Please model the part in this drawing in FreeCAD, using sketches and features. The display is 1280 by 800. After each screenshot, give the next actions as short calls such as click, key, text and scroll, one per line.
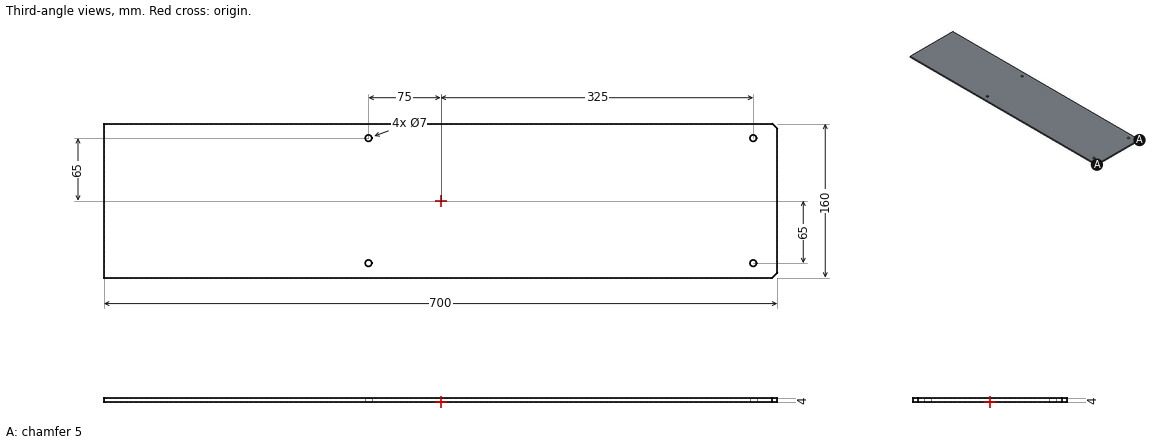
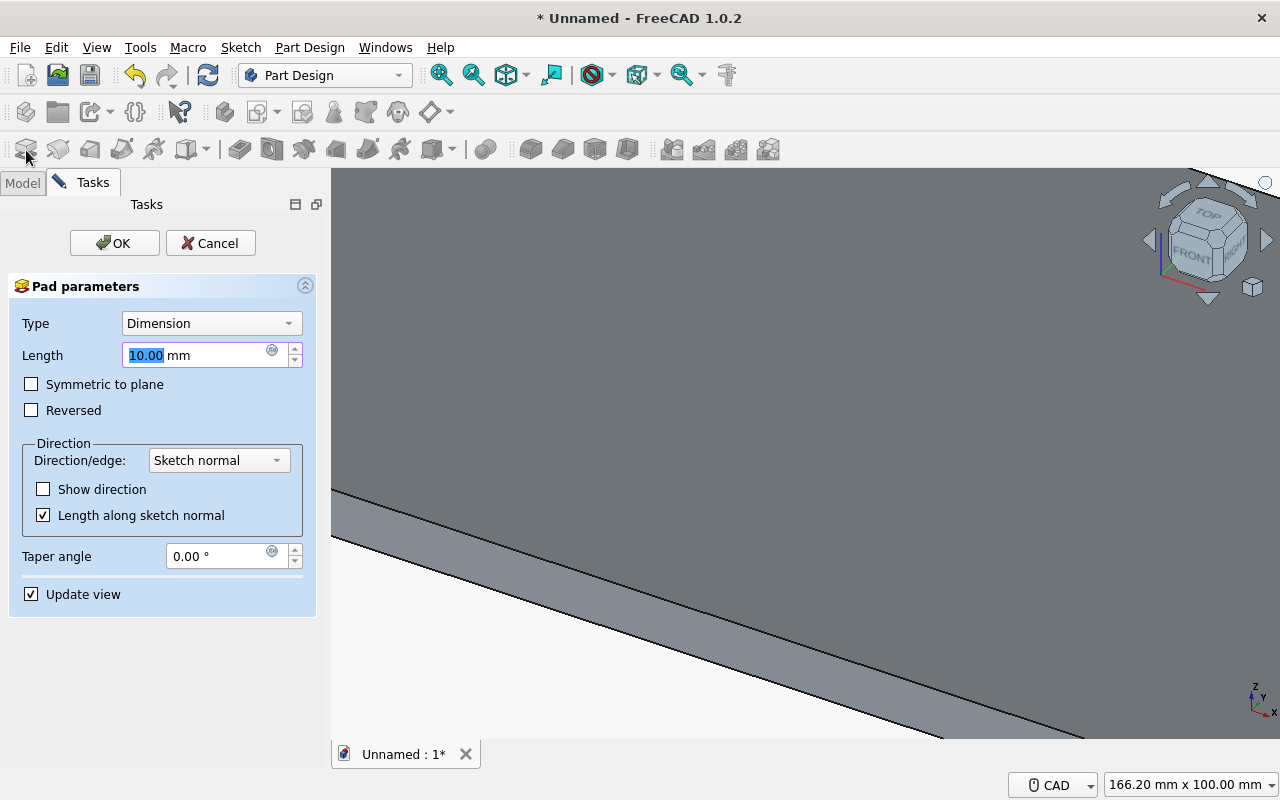
text(4)
key(Tab)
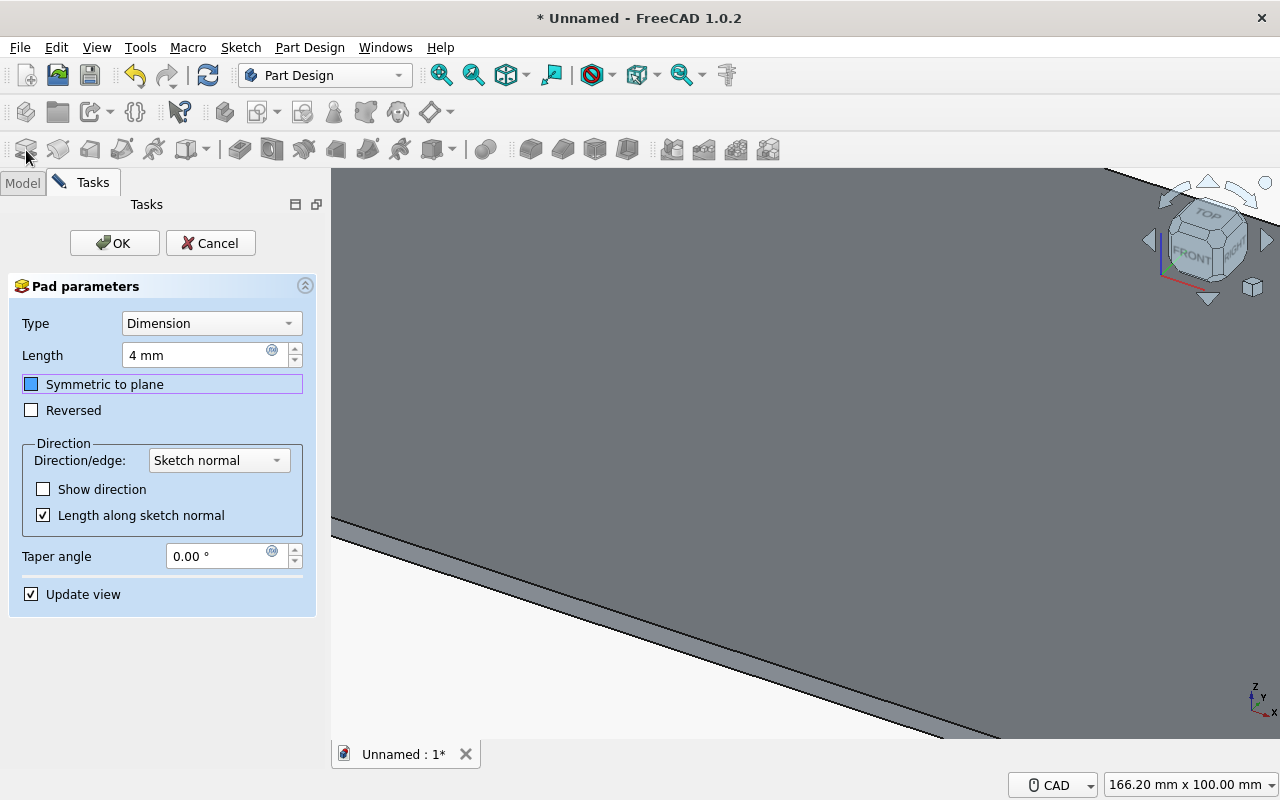
click(115, 243)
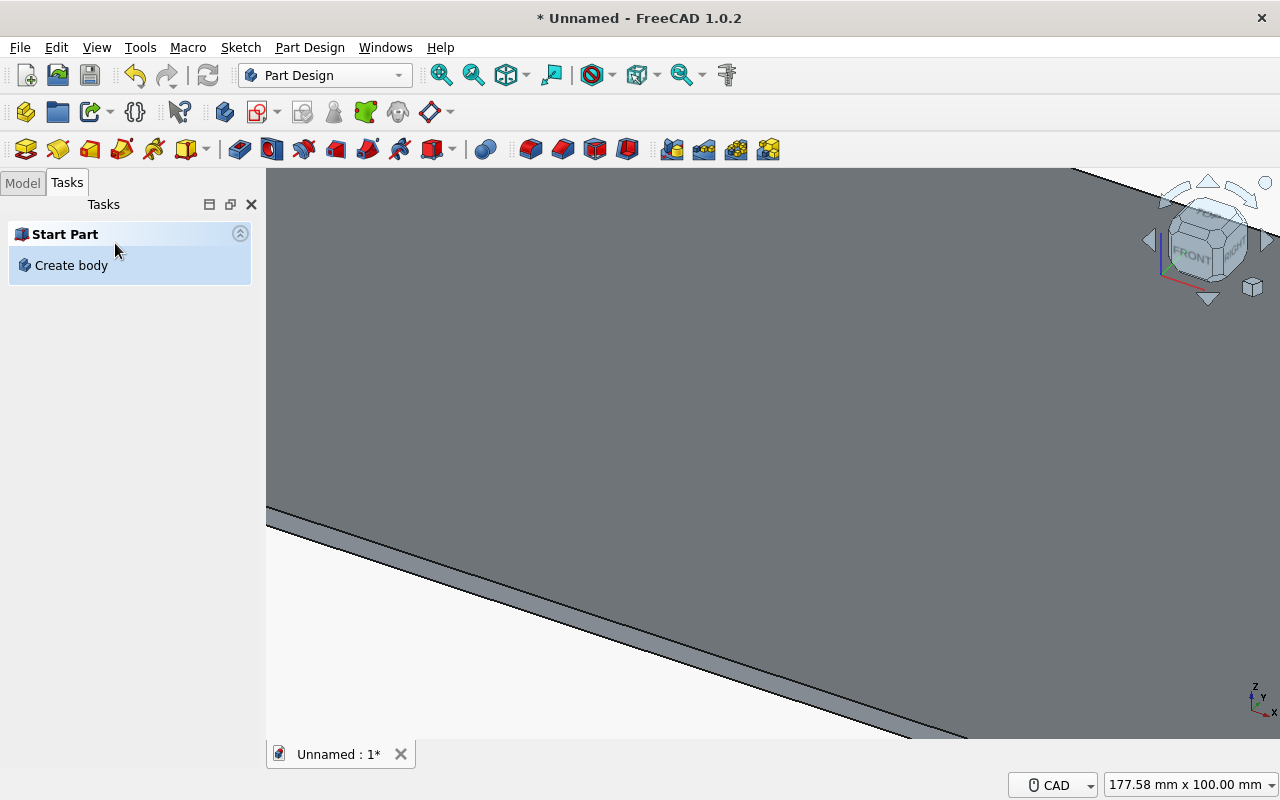
click(442, 76)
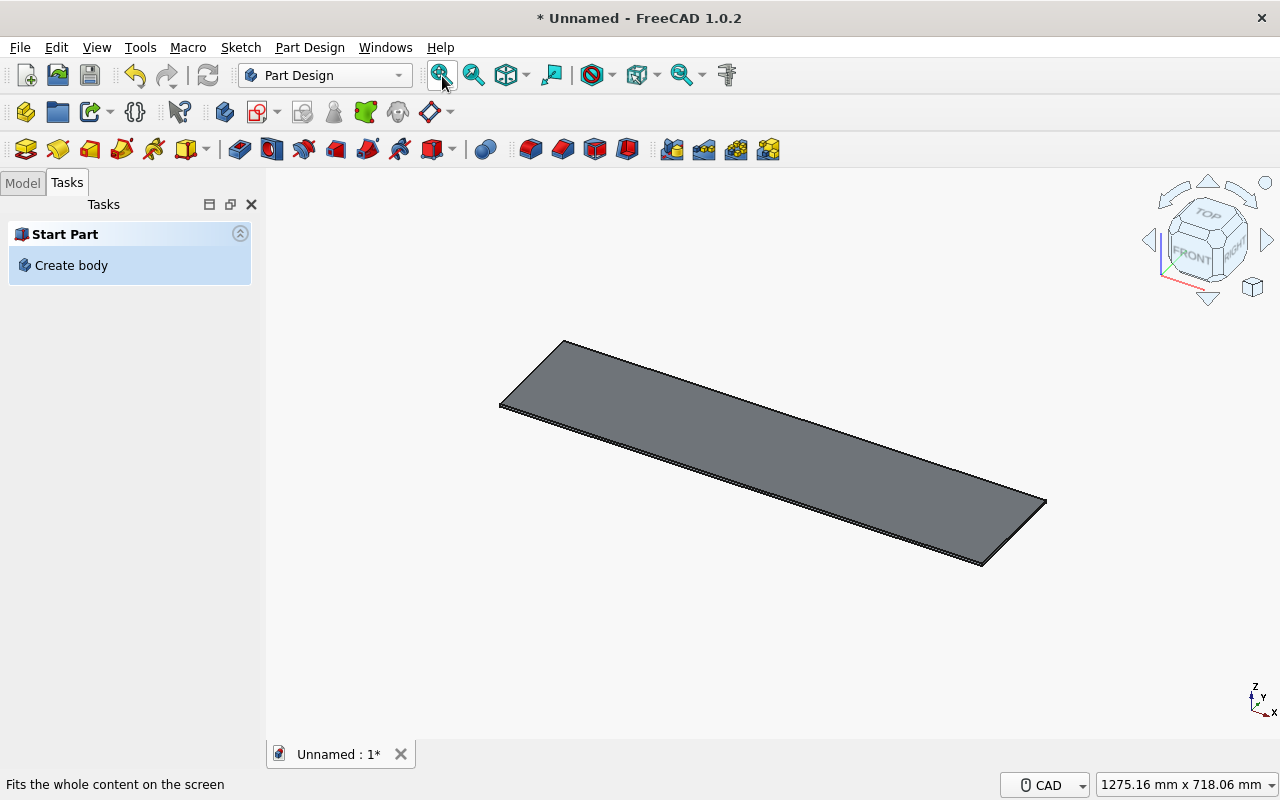
click(911, 497)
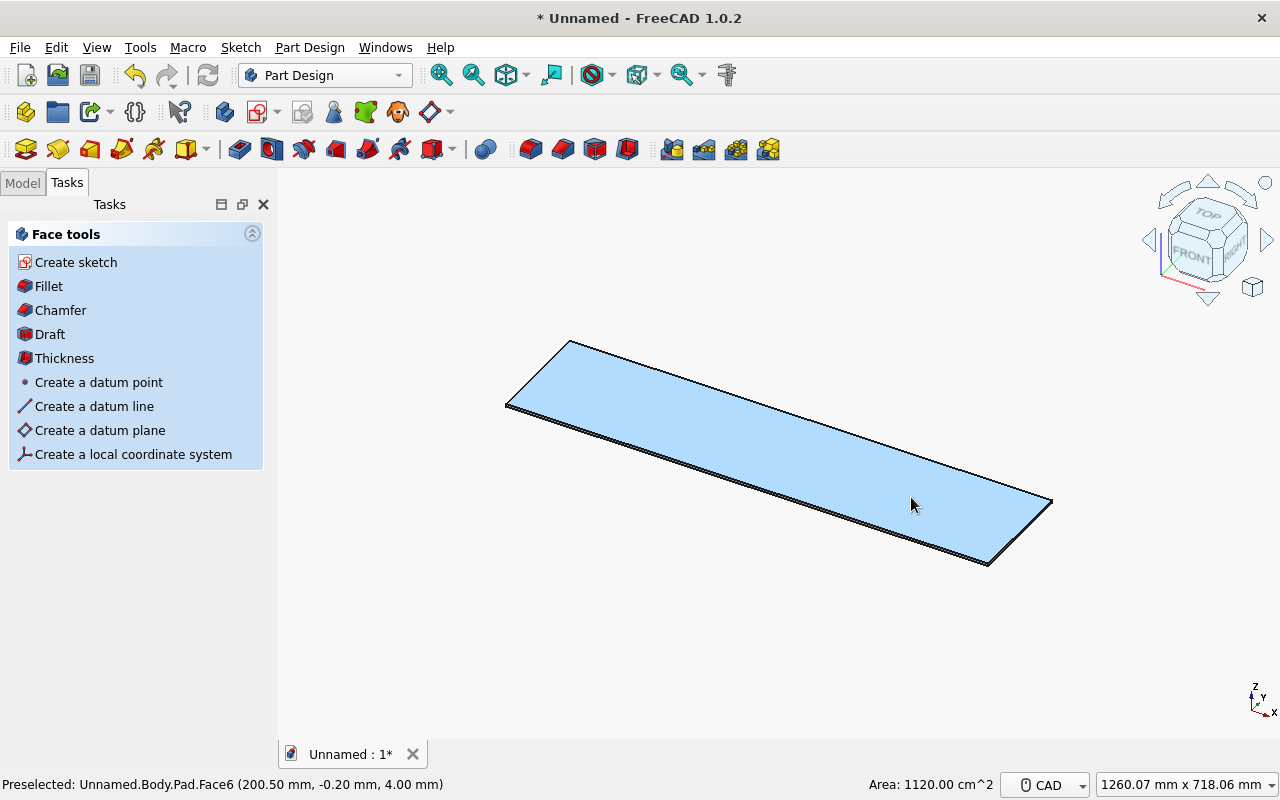
click(258, 112)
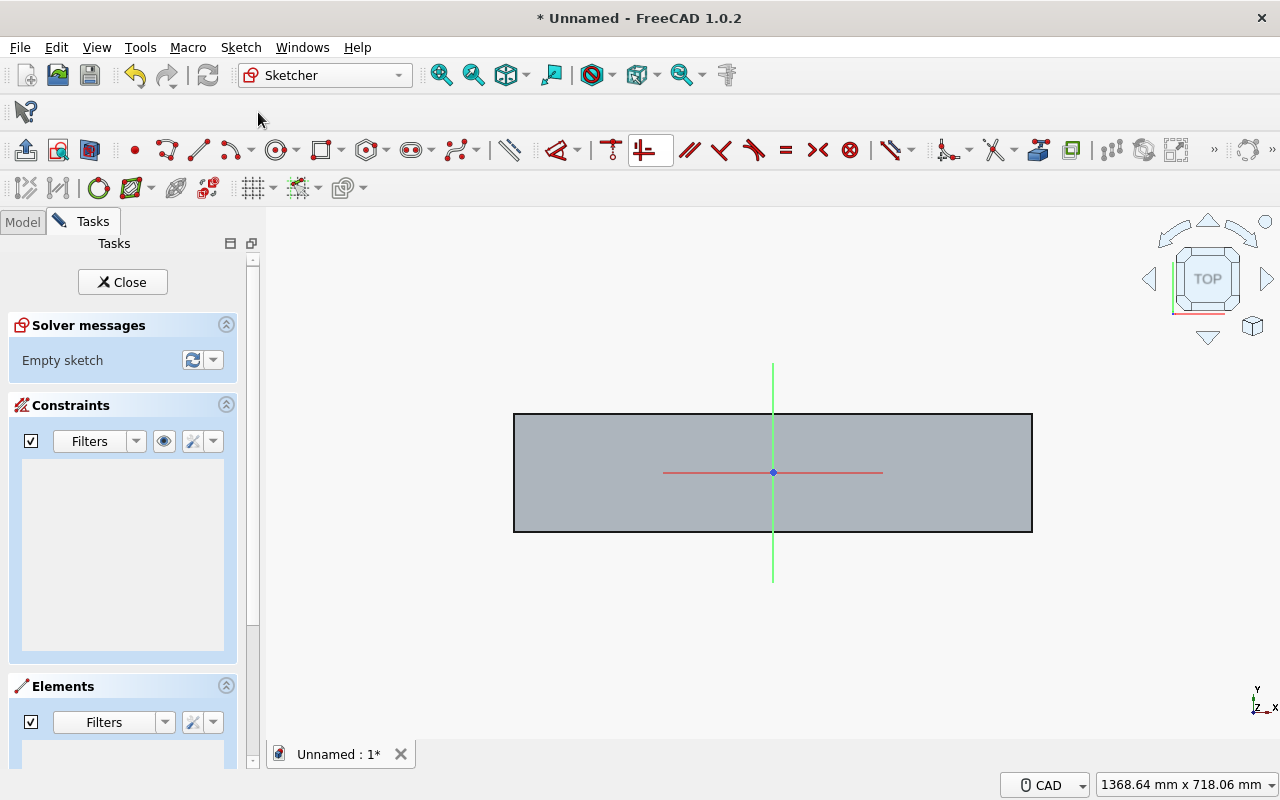
scroll(1062, 473, up, 3)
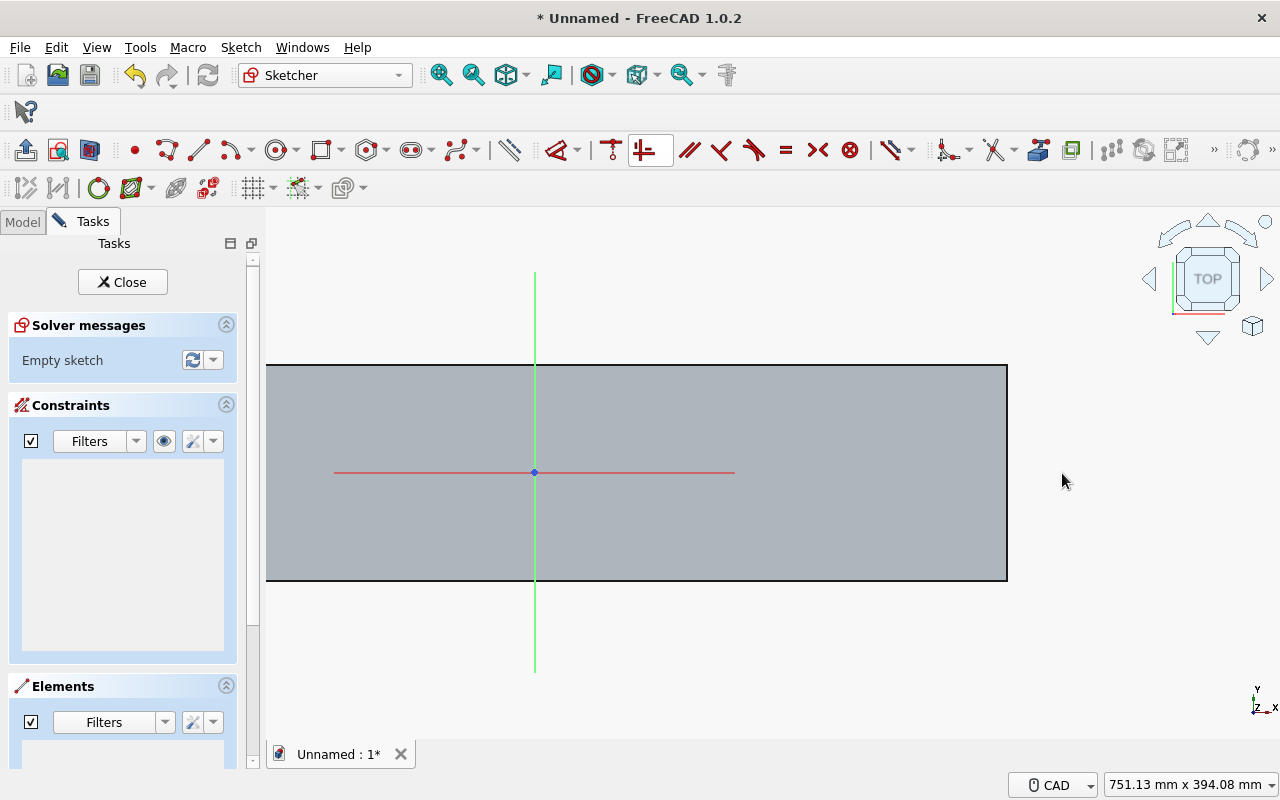
click(276, 150)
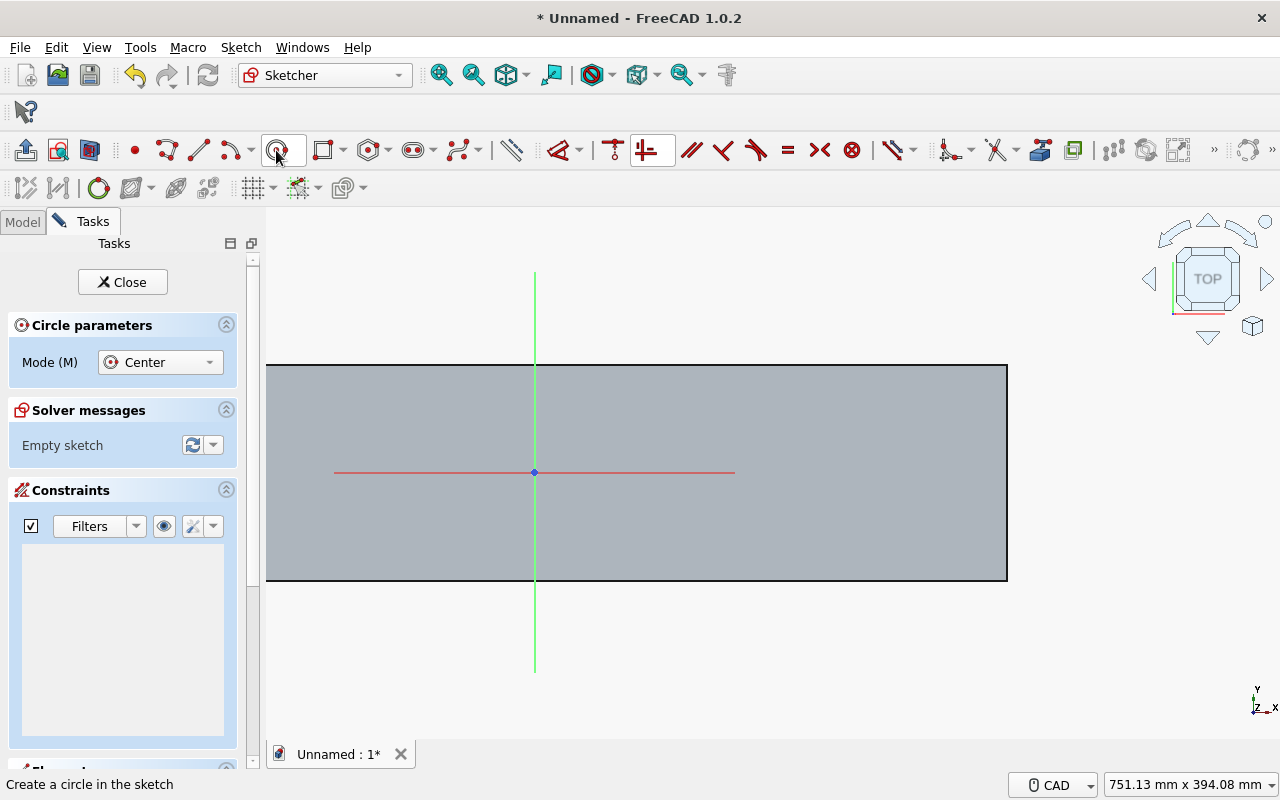
scroll(434, 385, up, 8)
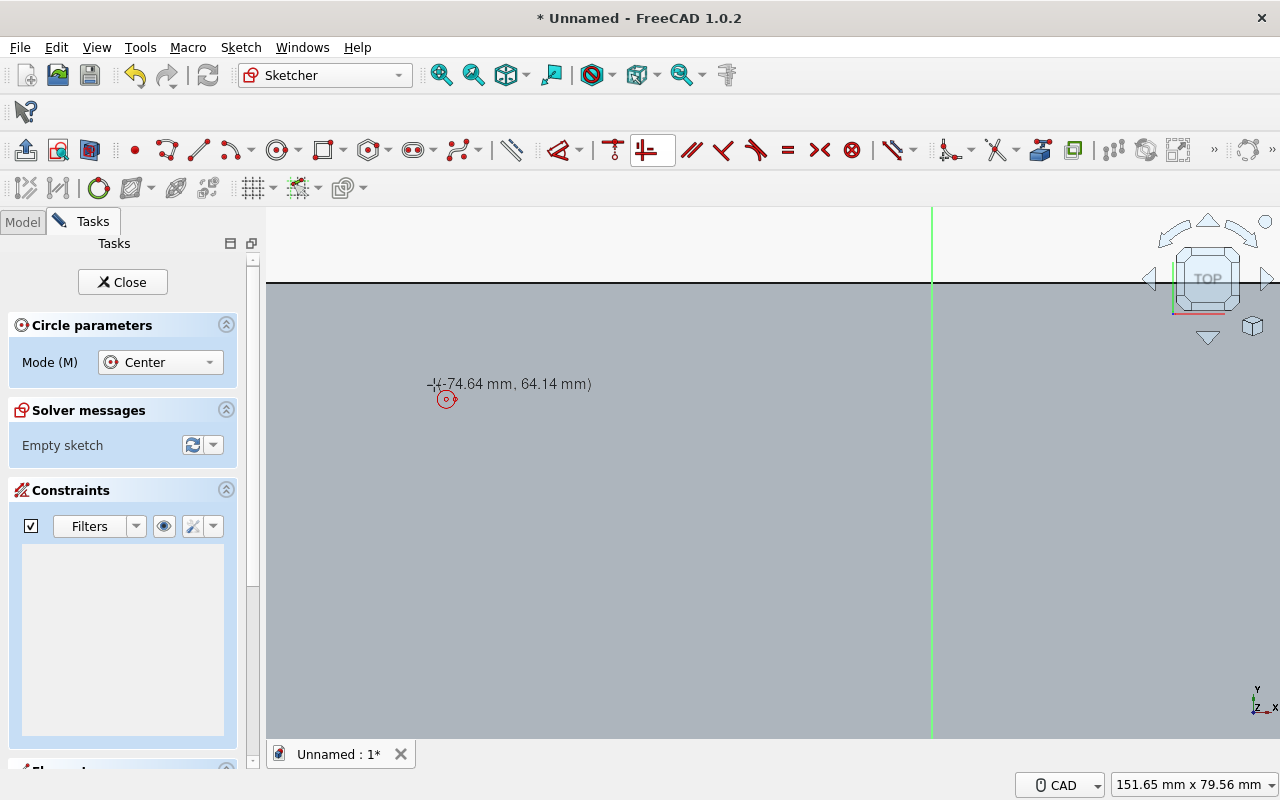
scroll(435, 386, down, 8)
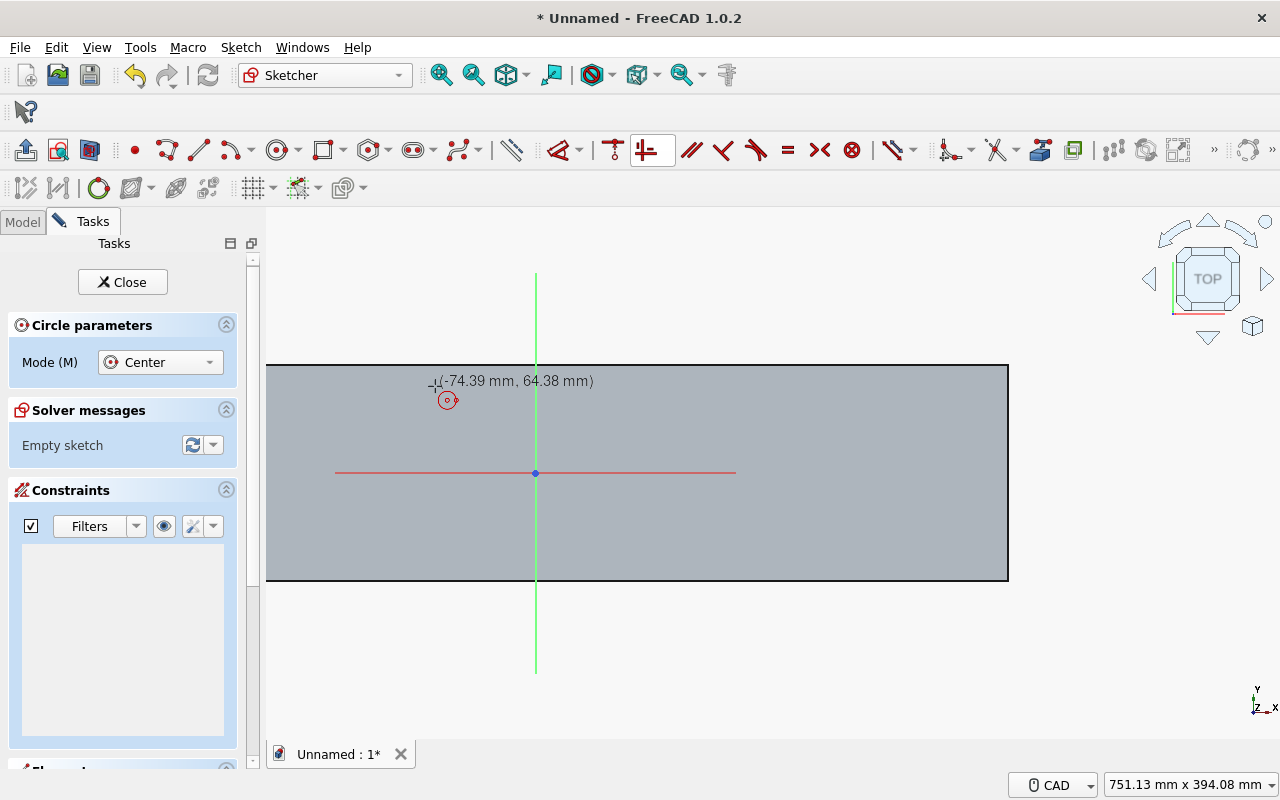
click(434, 386)
move(438, 382)